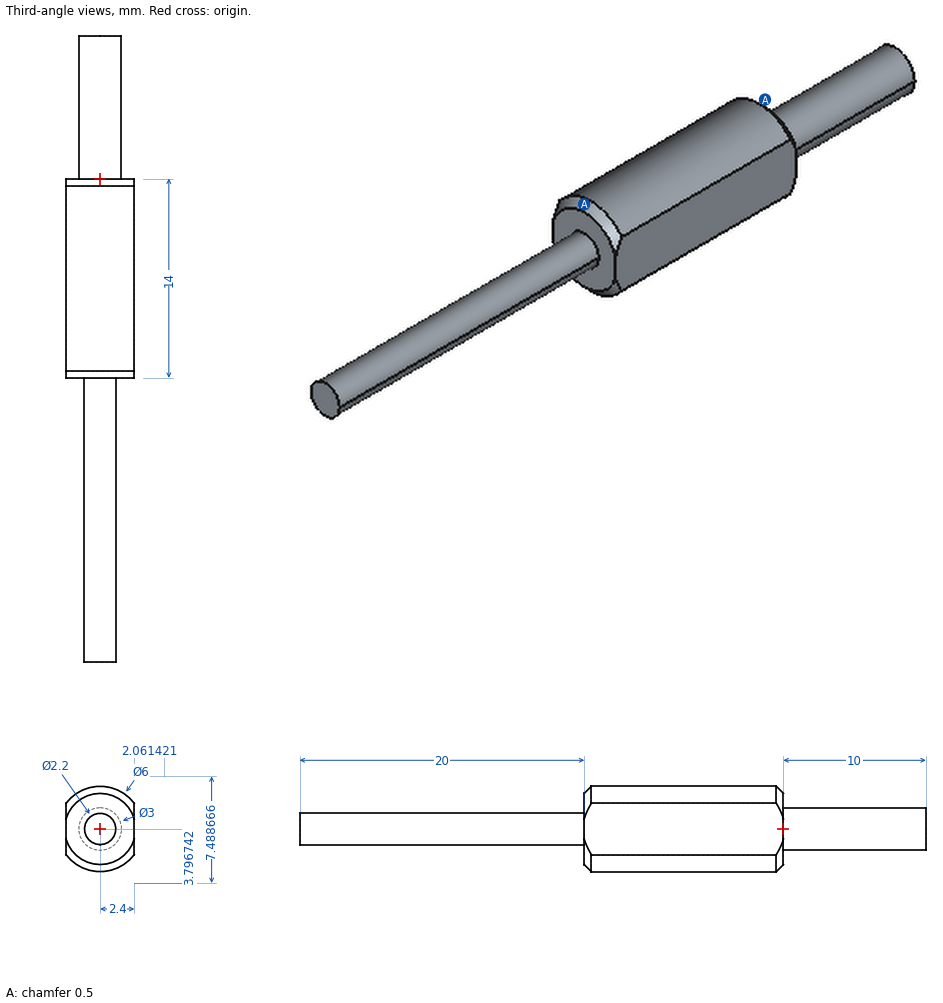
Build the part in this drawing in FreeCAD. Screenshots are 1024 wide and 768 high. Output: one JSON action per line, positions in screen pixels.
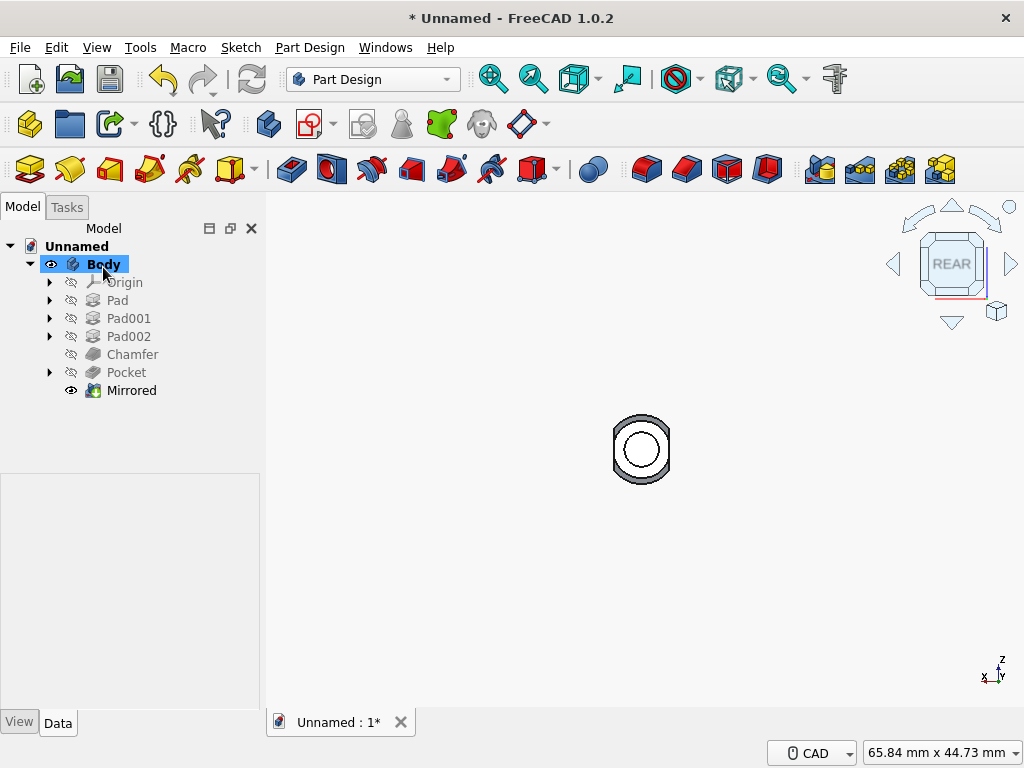
{"action": "key", "text": "0"}